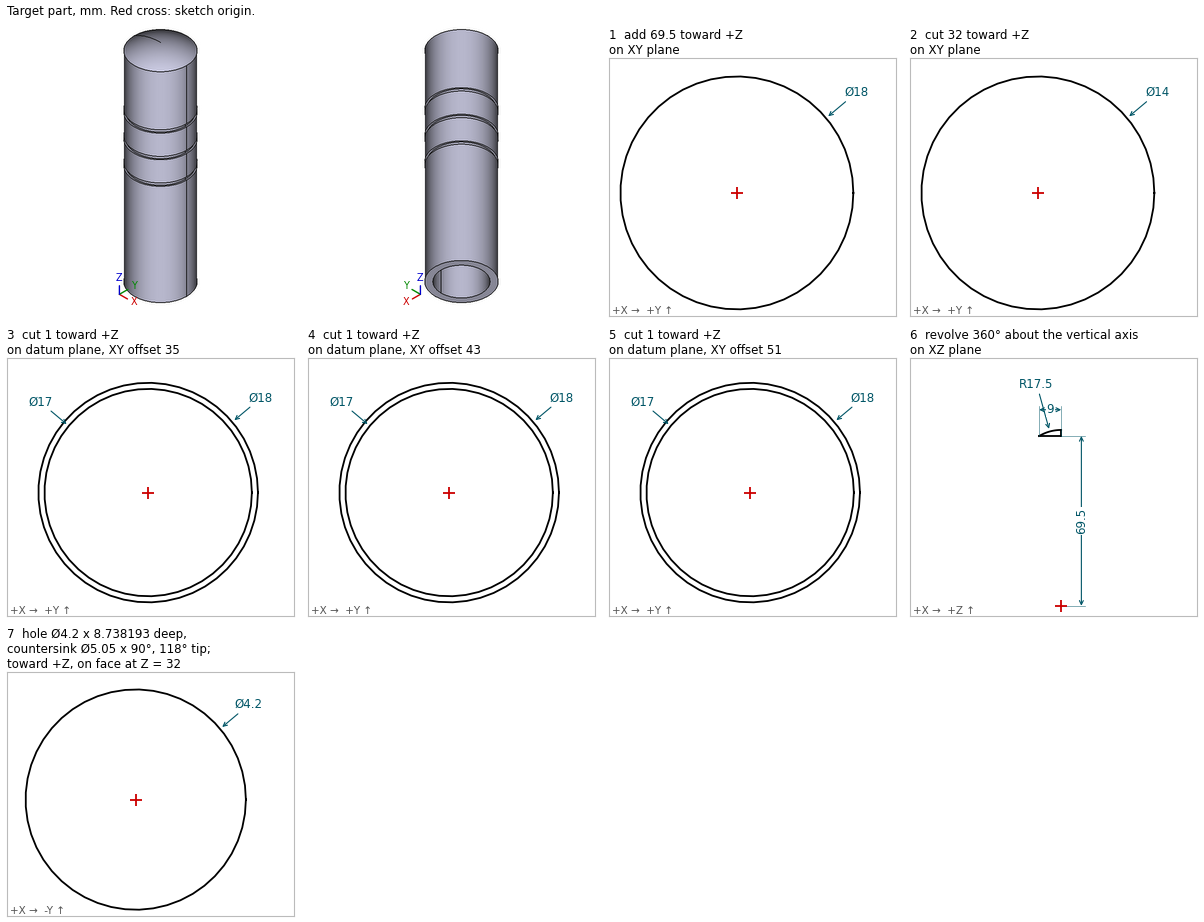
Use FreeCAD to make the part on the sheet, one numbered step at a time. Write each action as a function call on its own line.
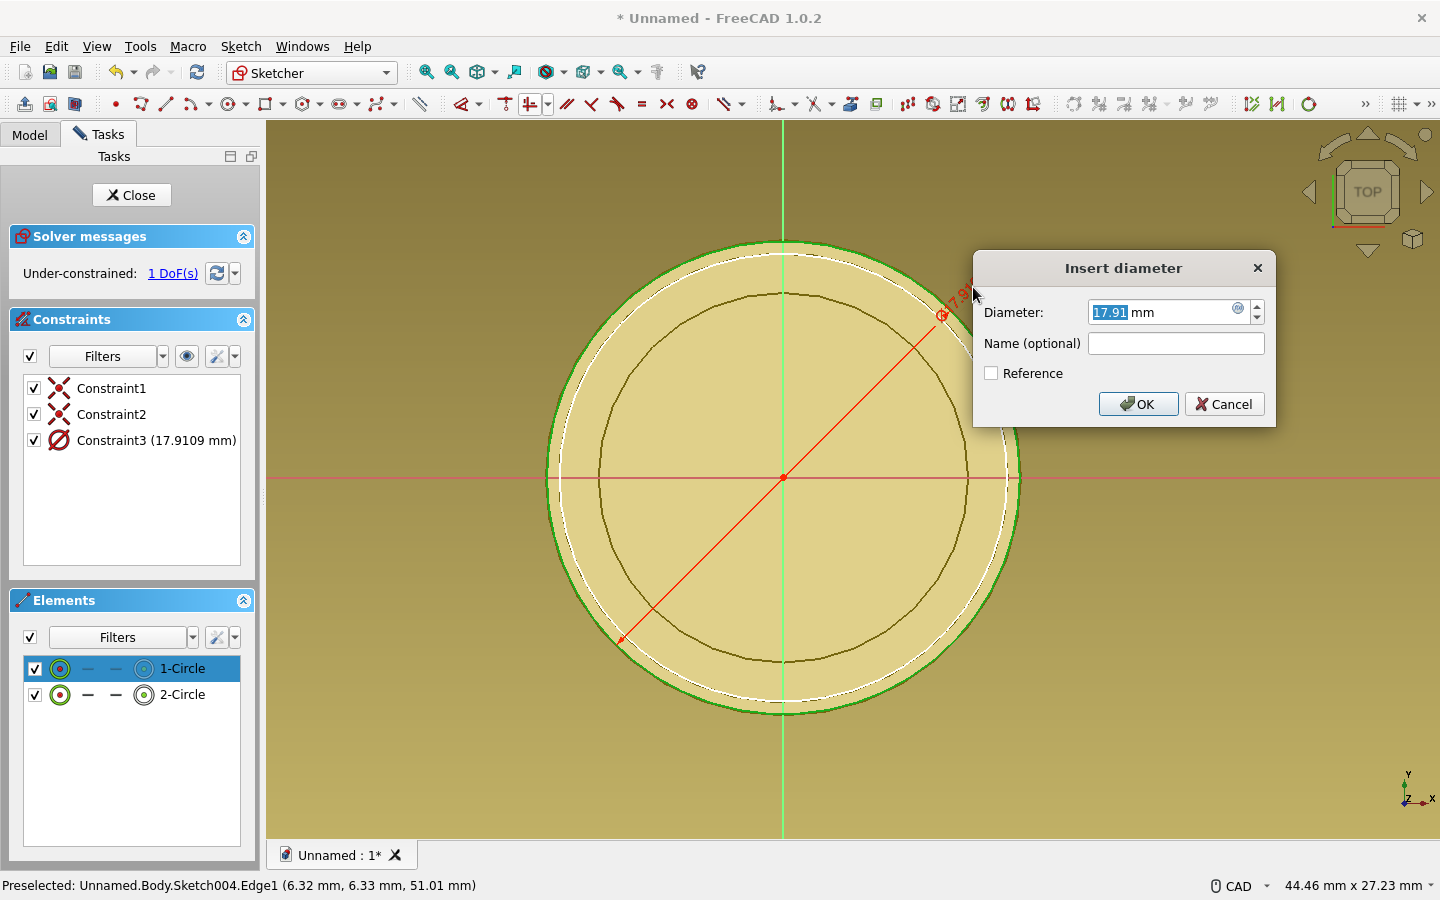
text(18)
key(Return)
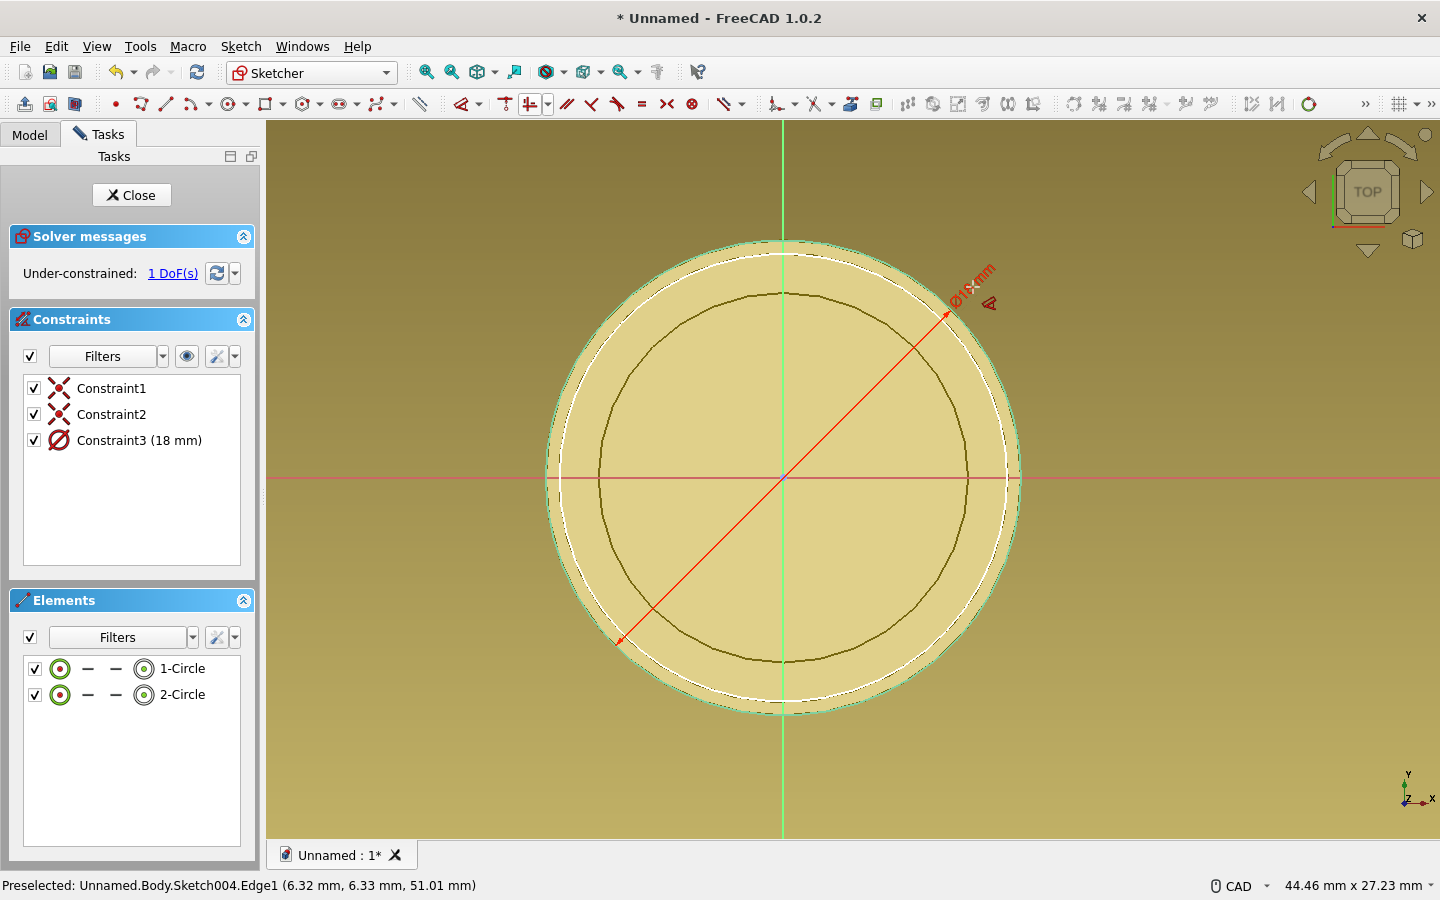
click(941, 319)
click(1028, 405)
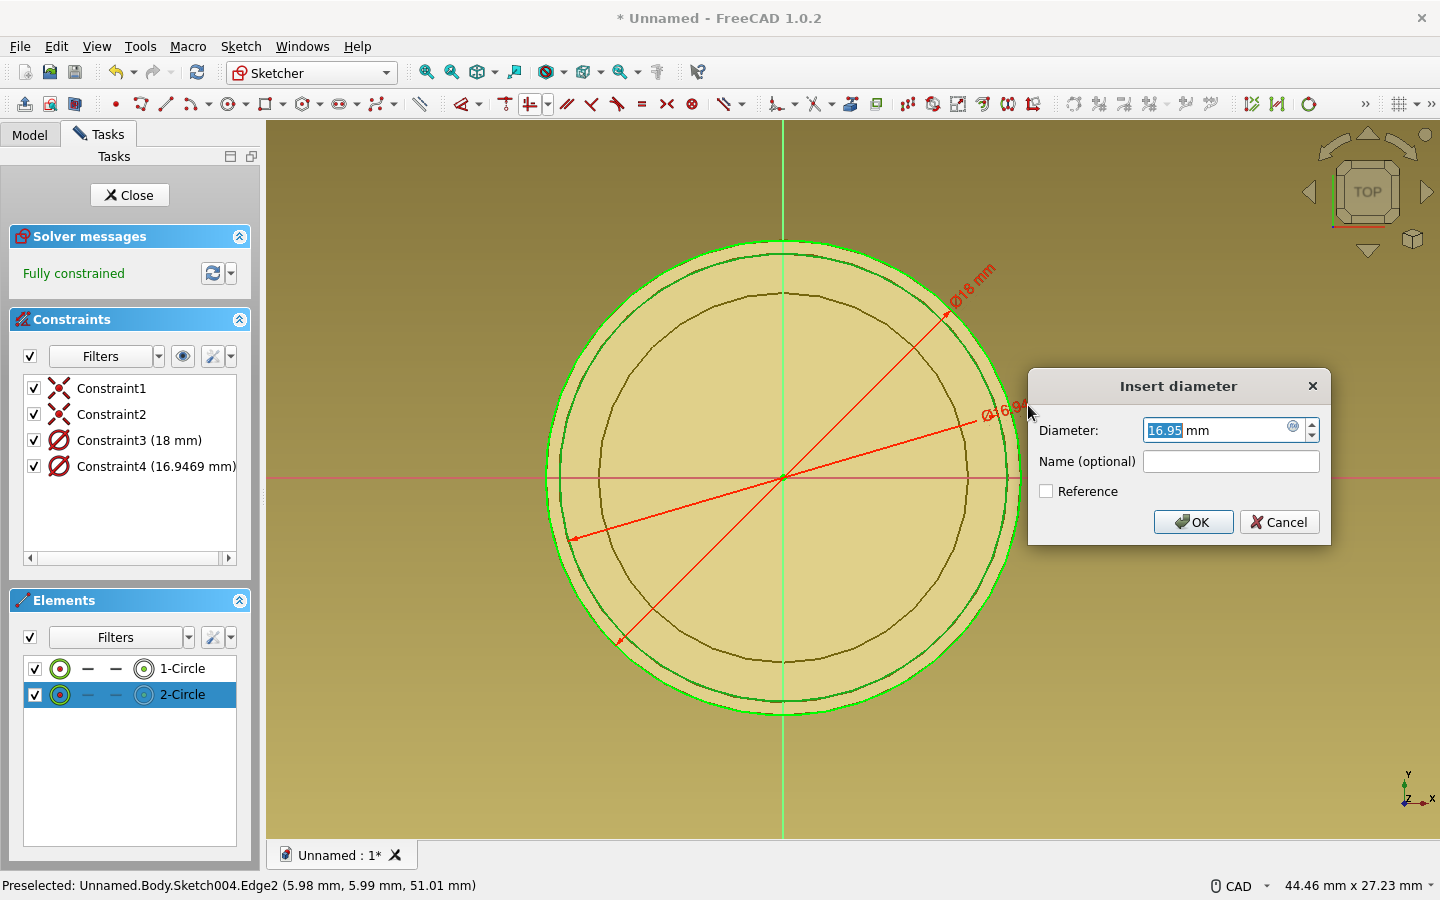
text(17)
key(Return)
key(Escape)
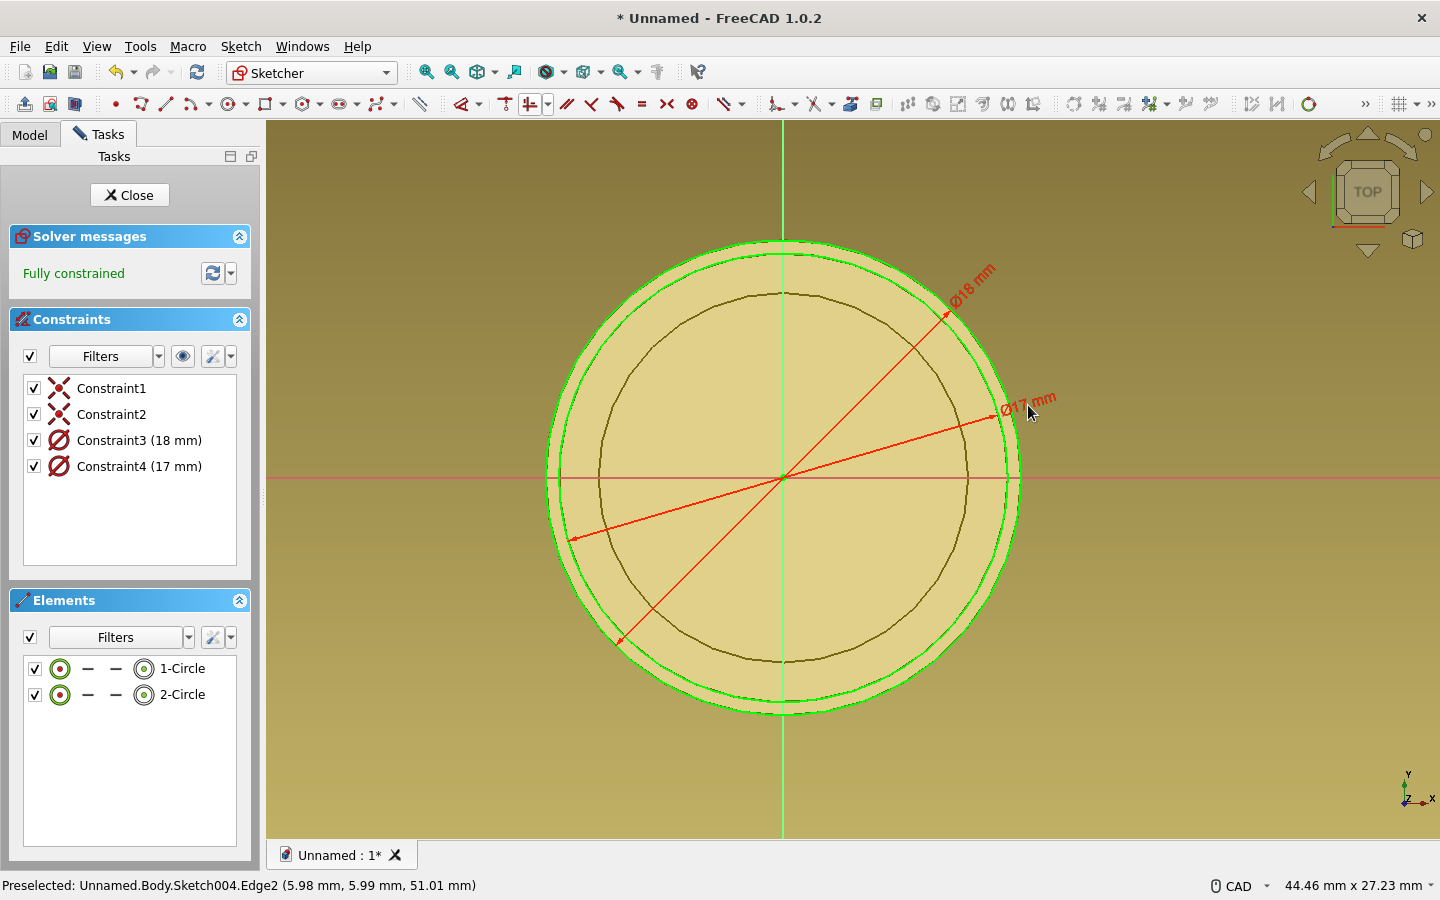
click(130, 195)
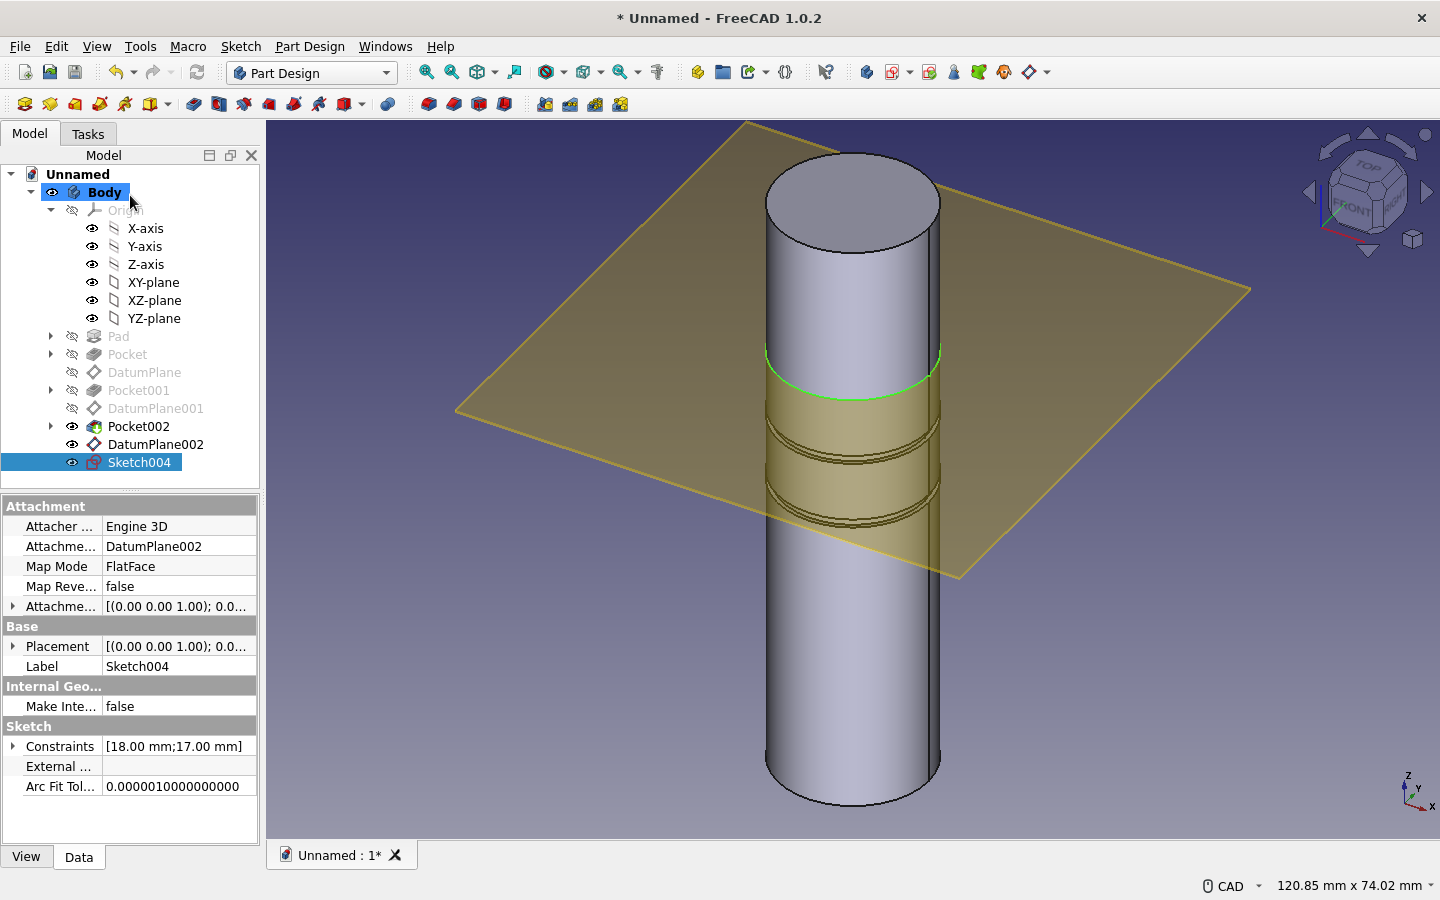
click(194, 104)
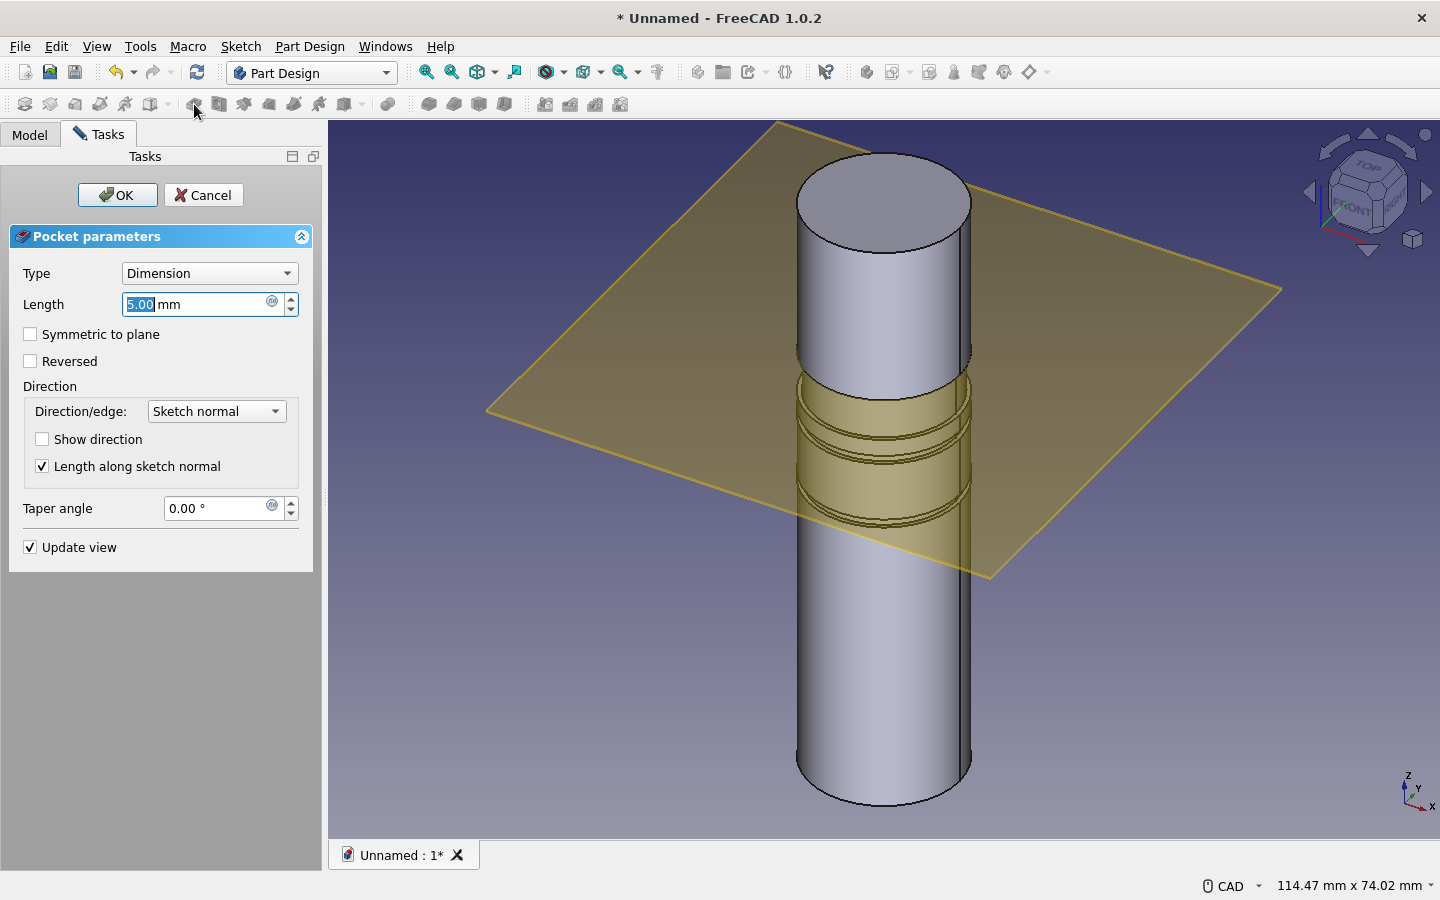
text(1)
key(Tab)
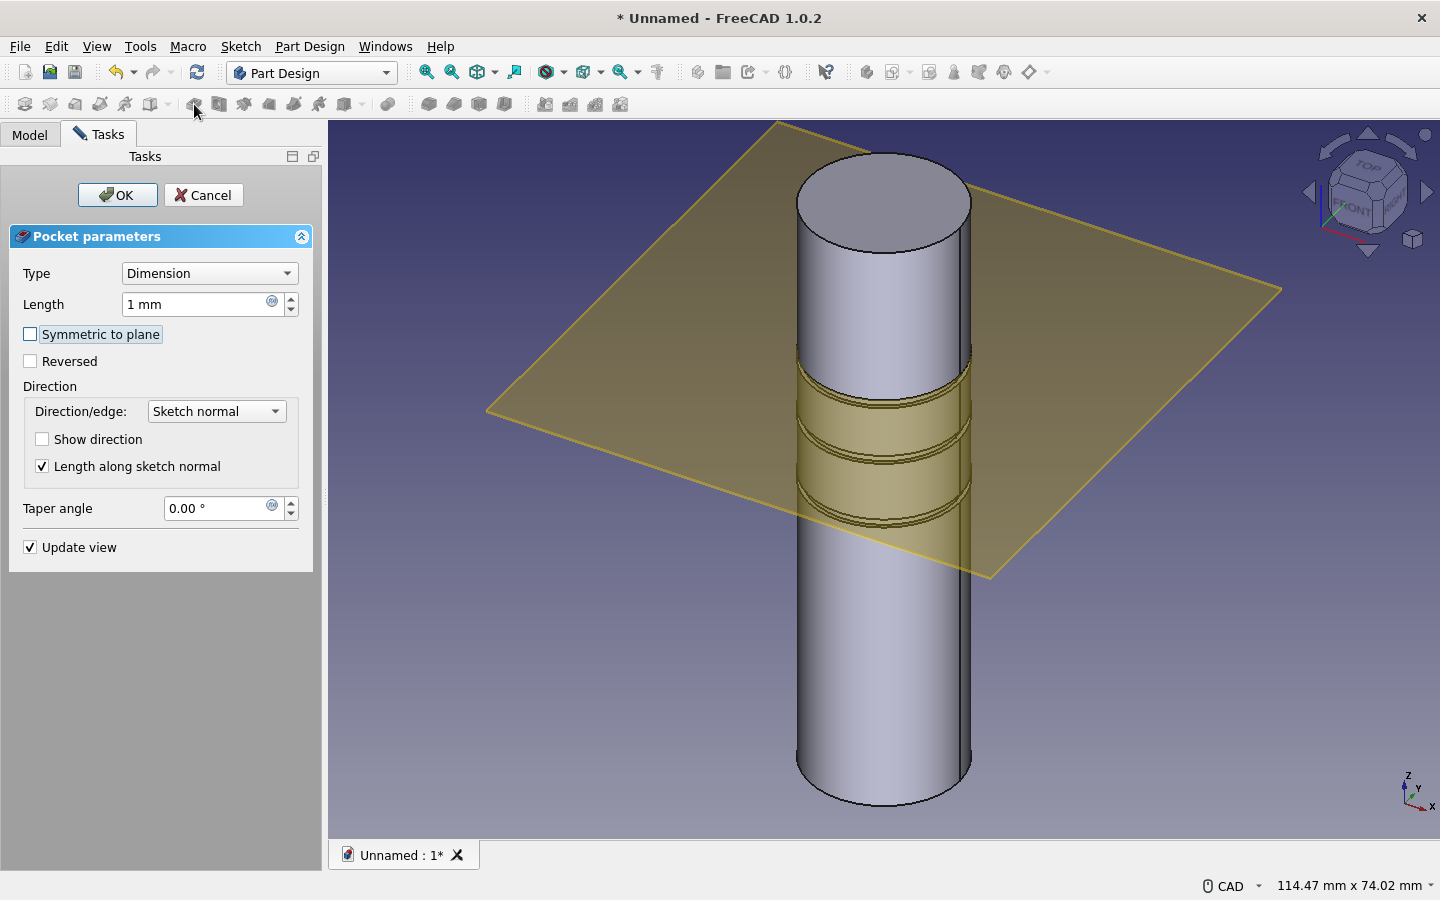
click(31, 361)